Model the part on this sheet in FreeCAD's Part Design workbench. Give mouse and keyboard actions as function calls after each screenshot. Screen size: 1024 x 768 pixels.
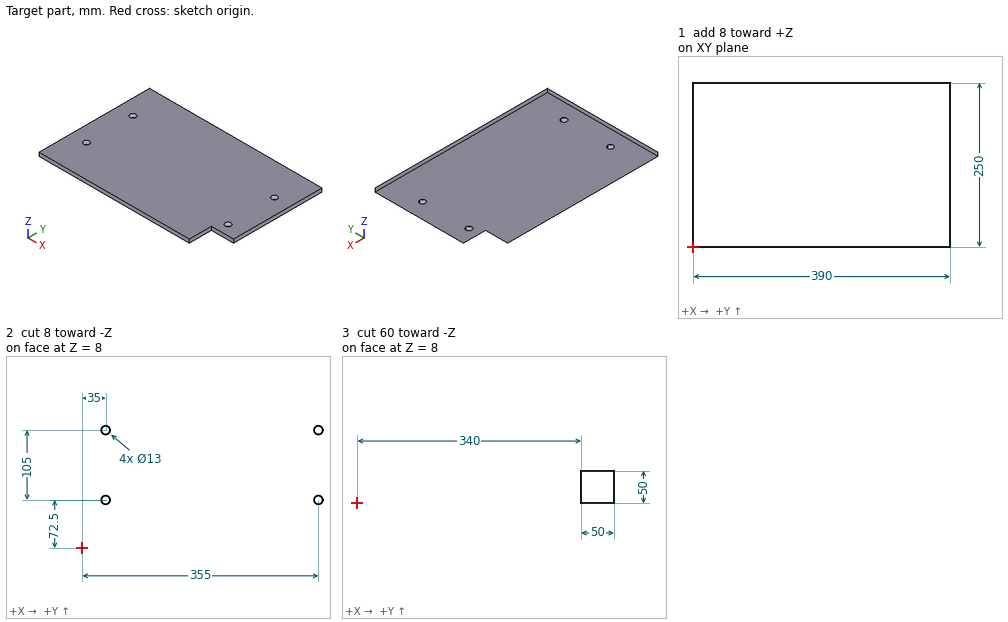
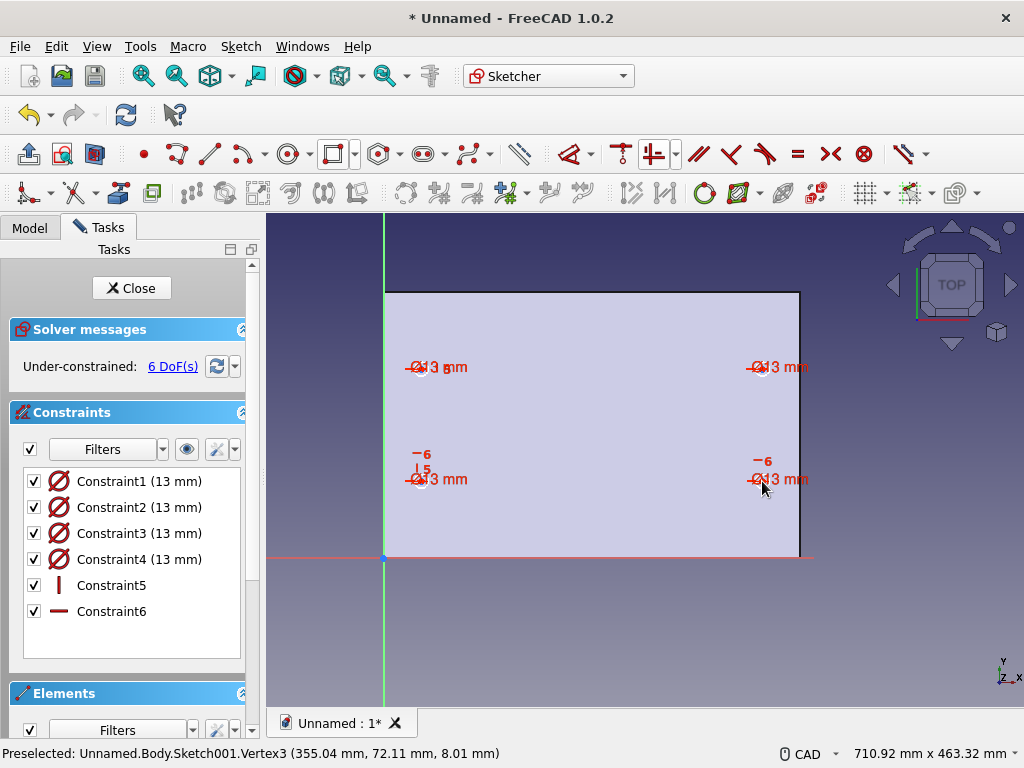
click(762, 481)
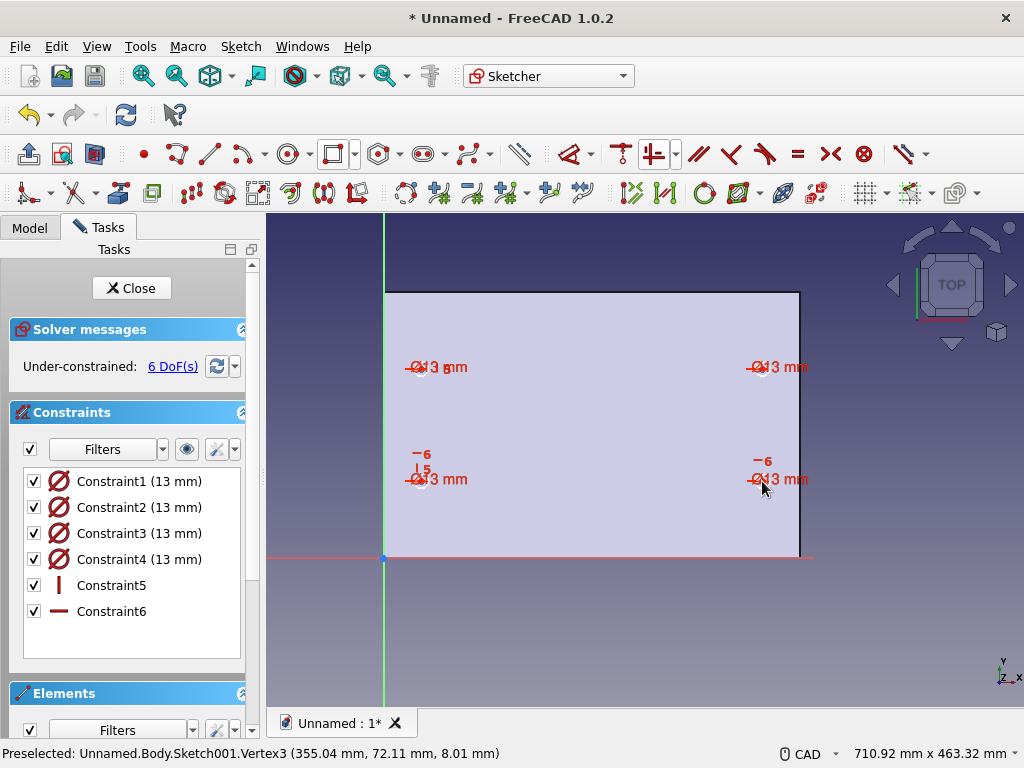
click(762, 369)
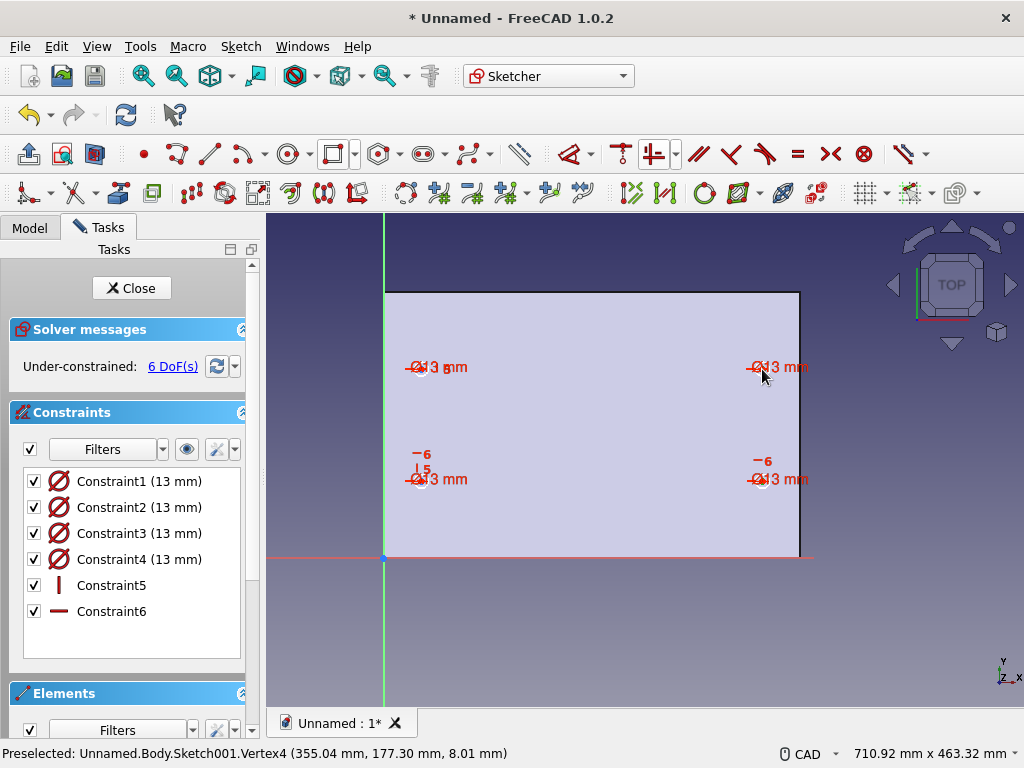
key(v)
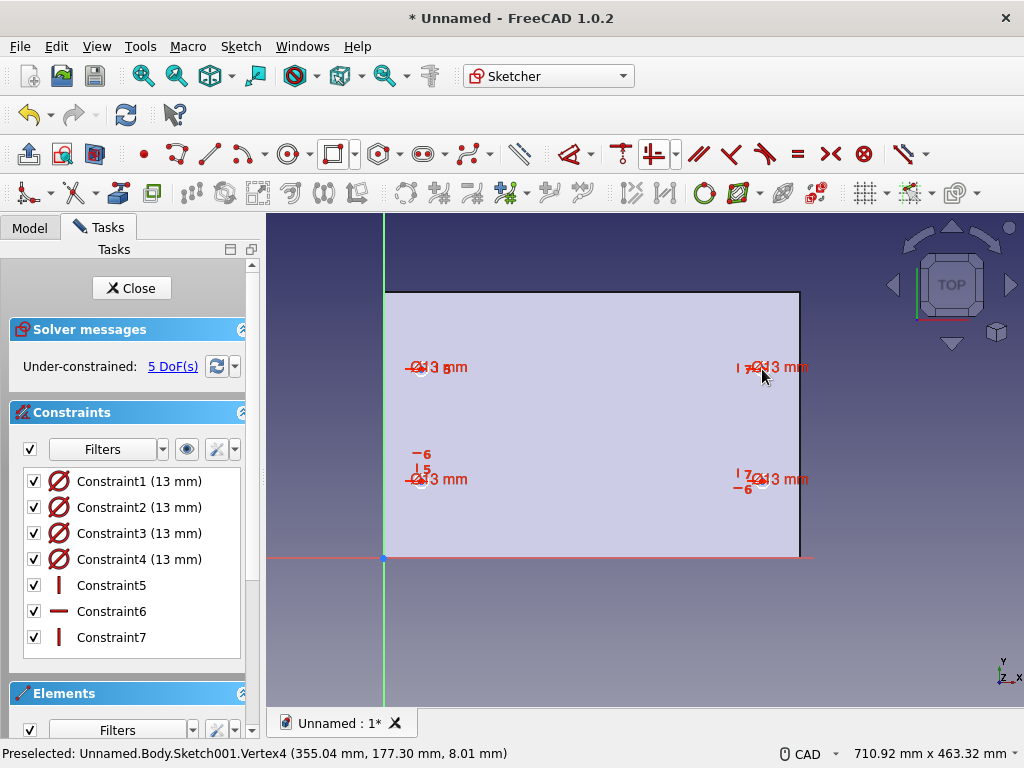
click(421, 369)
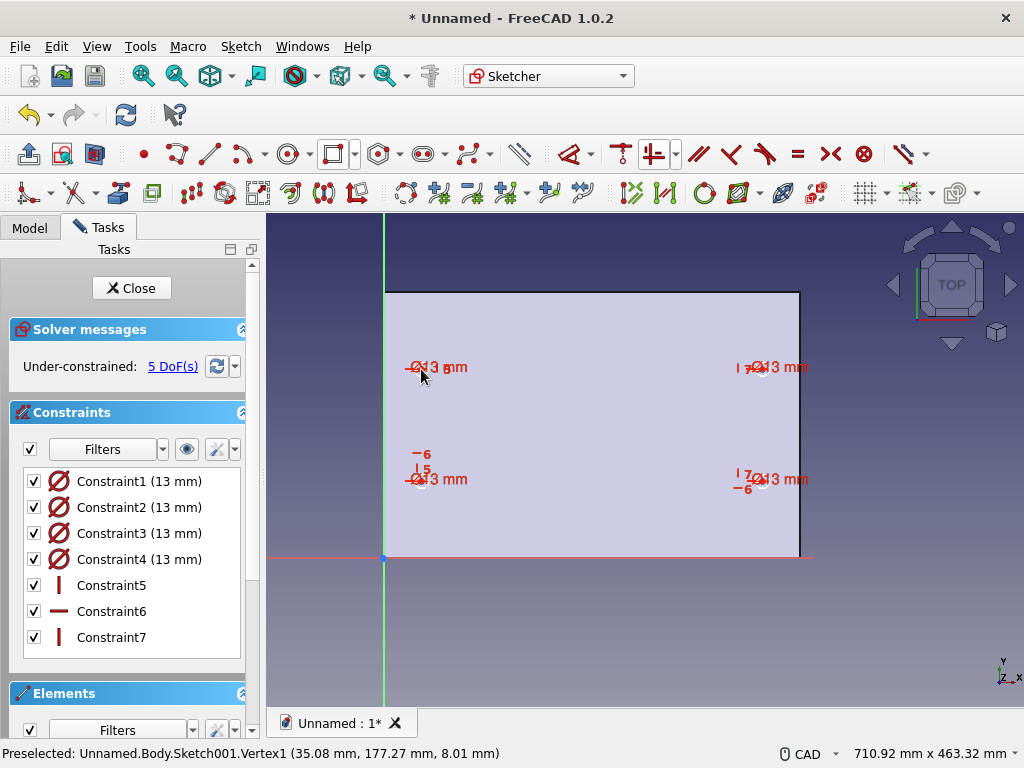
click(762, 369)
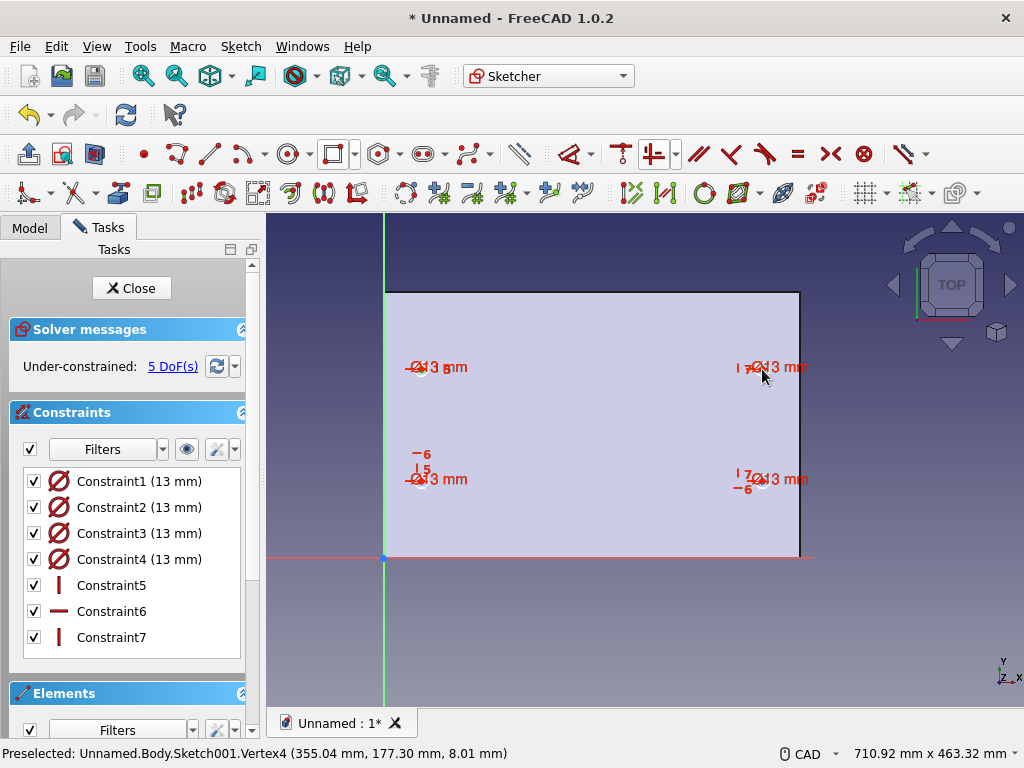
key(h)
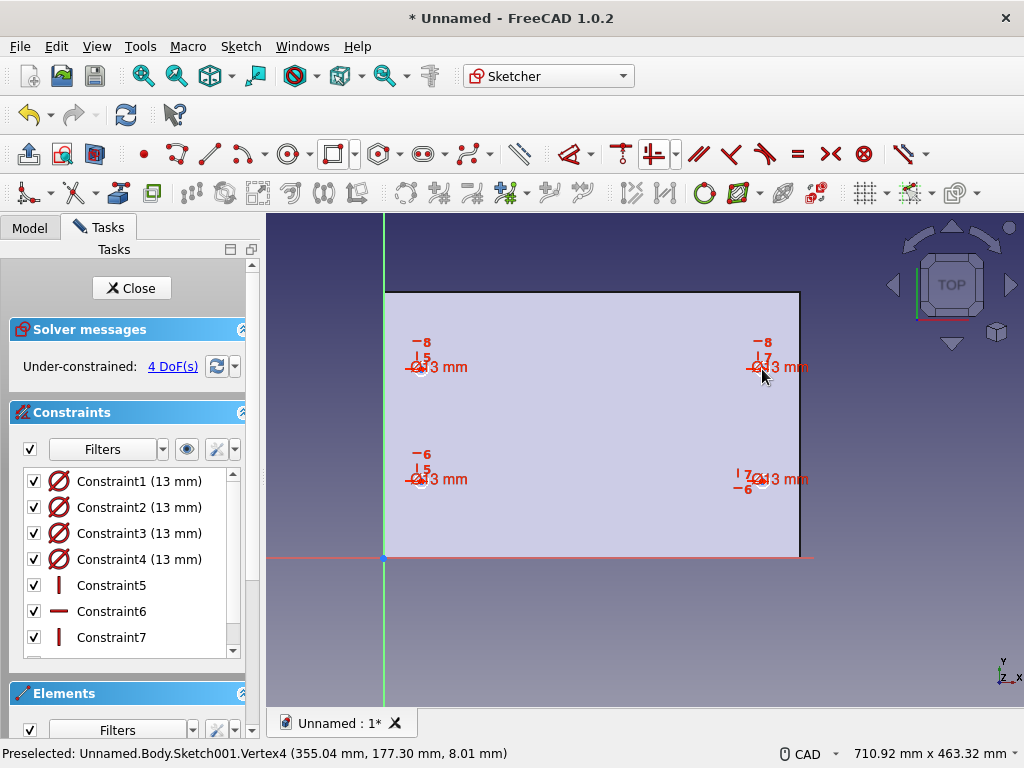
click(568, 154)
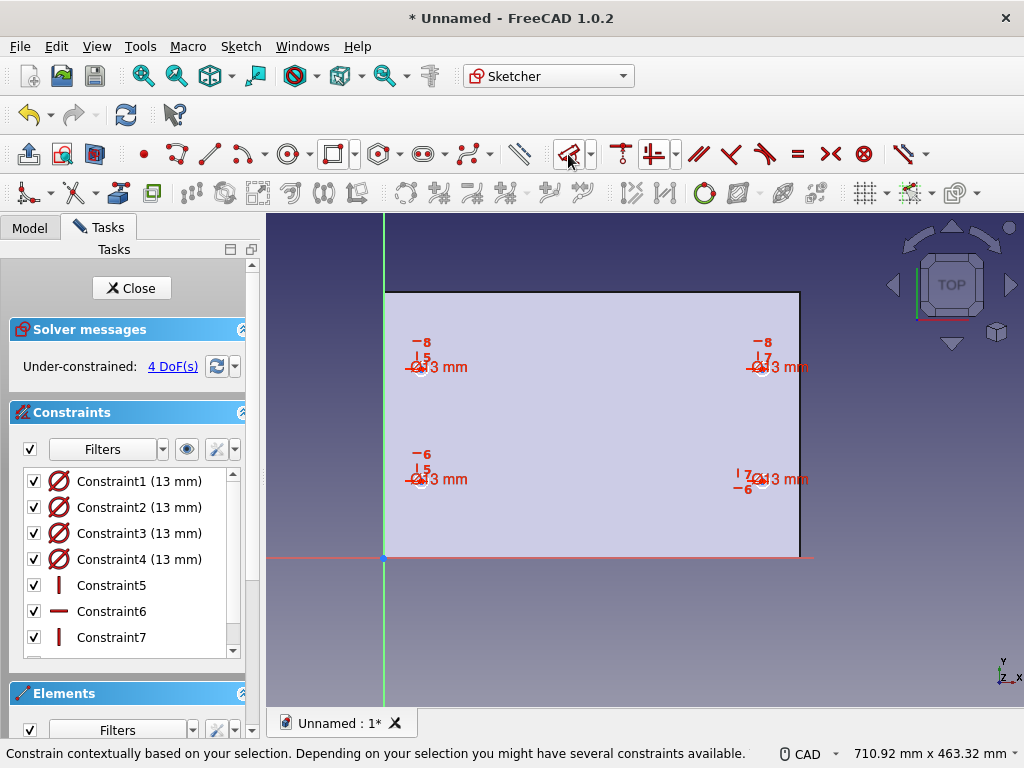
click(421, 369)
click(403, 592)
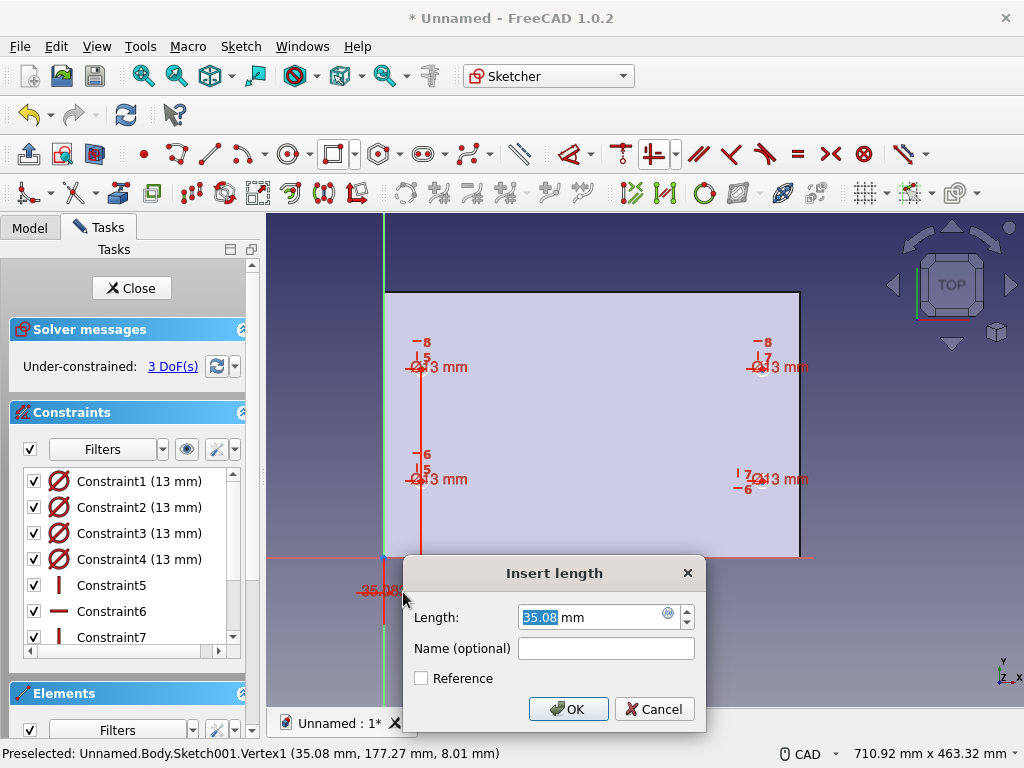
text(35)
key(Return)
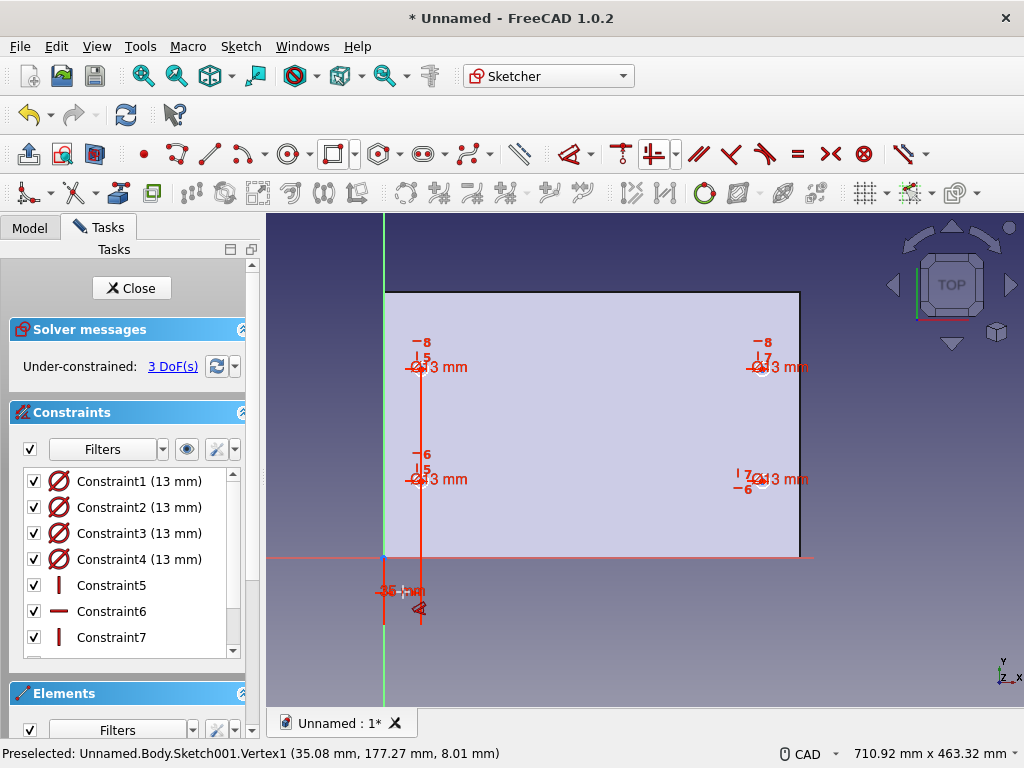
click(762, 481)
click(573, 592)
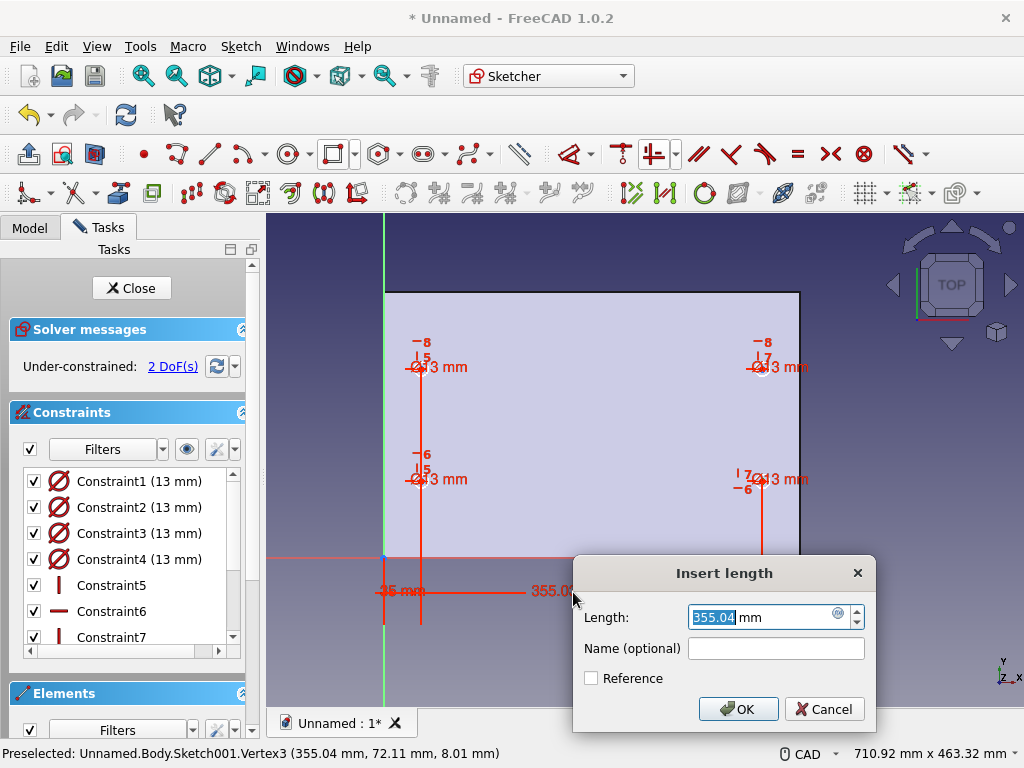
text(355)
key(Return)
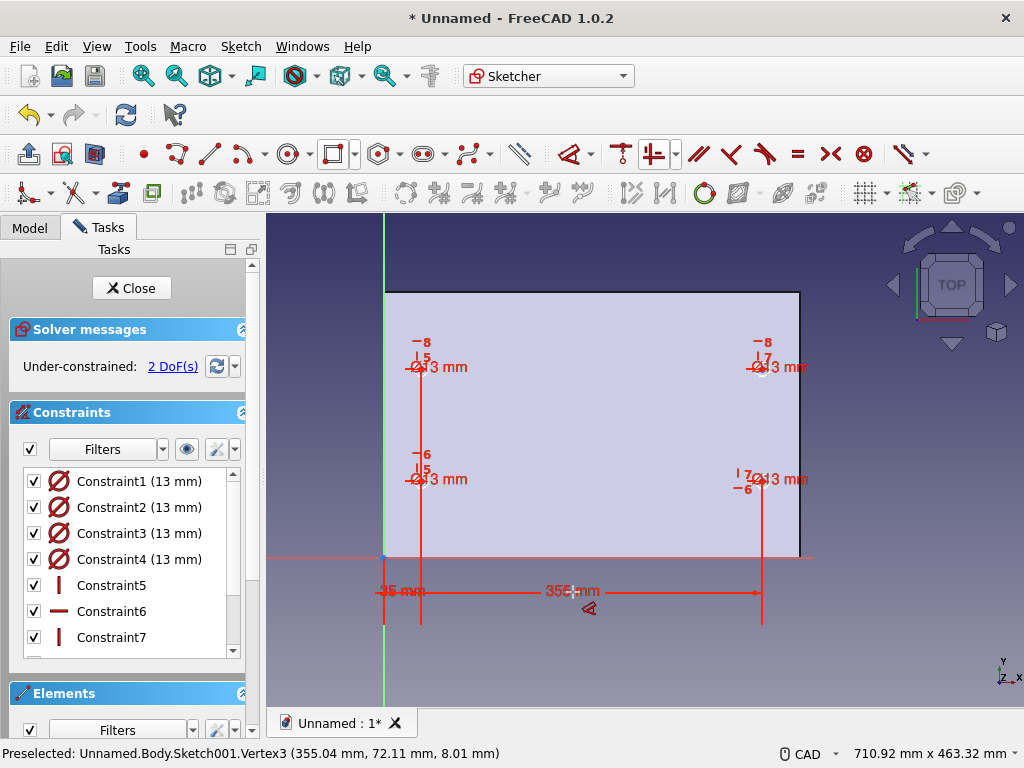
click(421, 481)
click(350, 520)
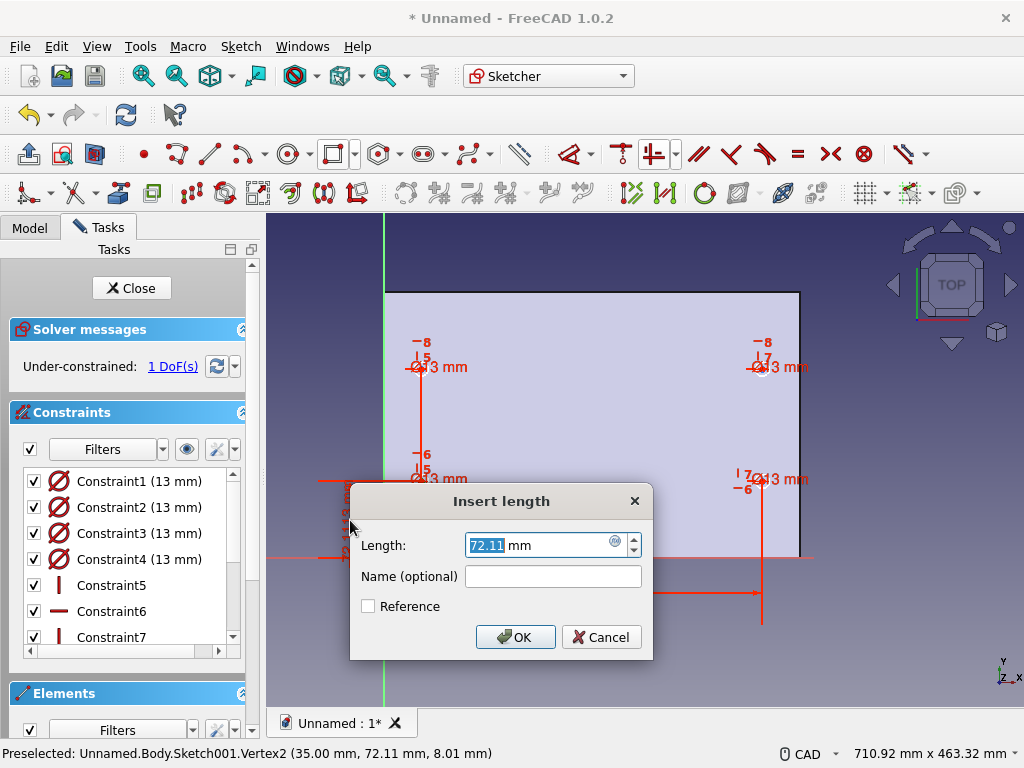
text(72.5)
key(Return)